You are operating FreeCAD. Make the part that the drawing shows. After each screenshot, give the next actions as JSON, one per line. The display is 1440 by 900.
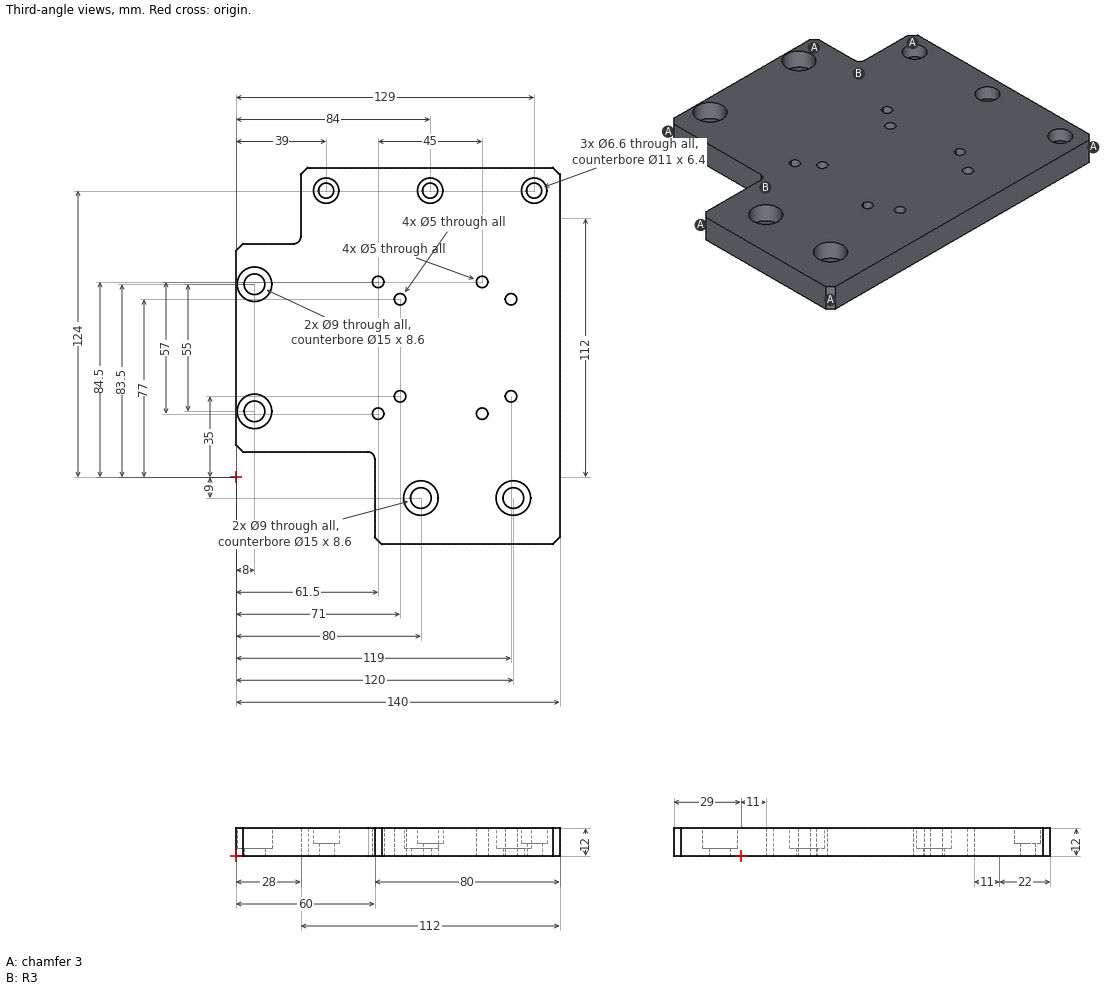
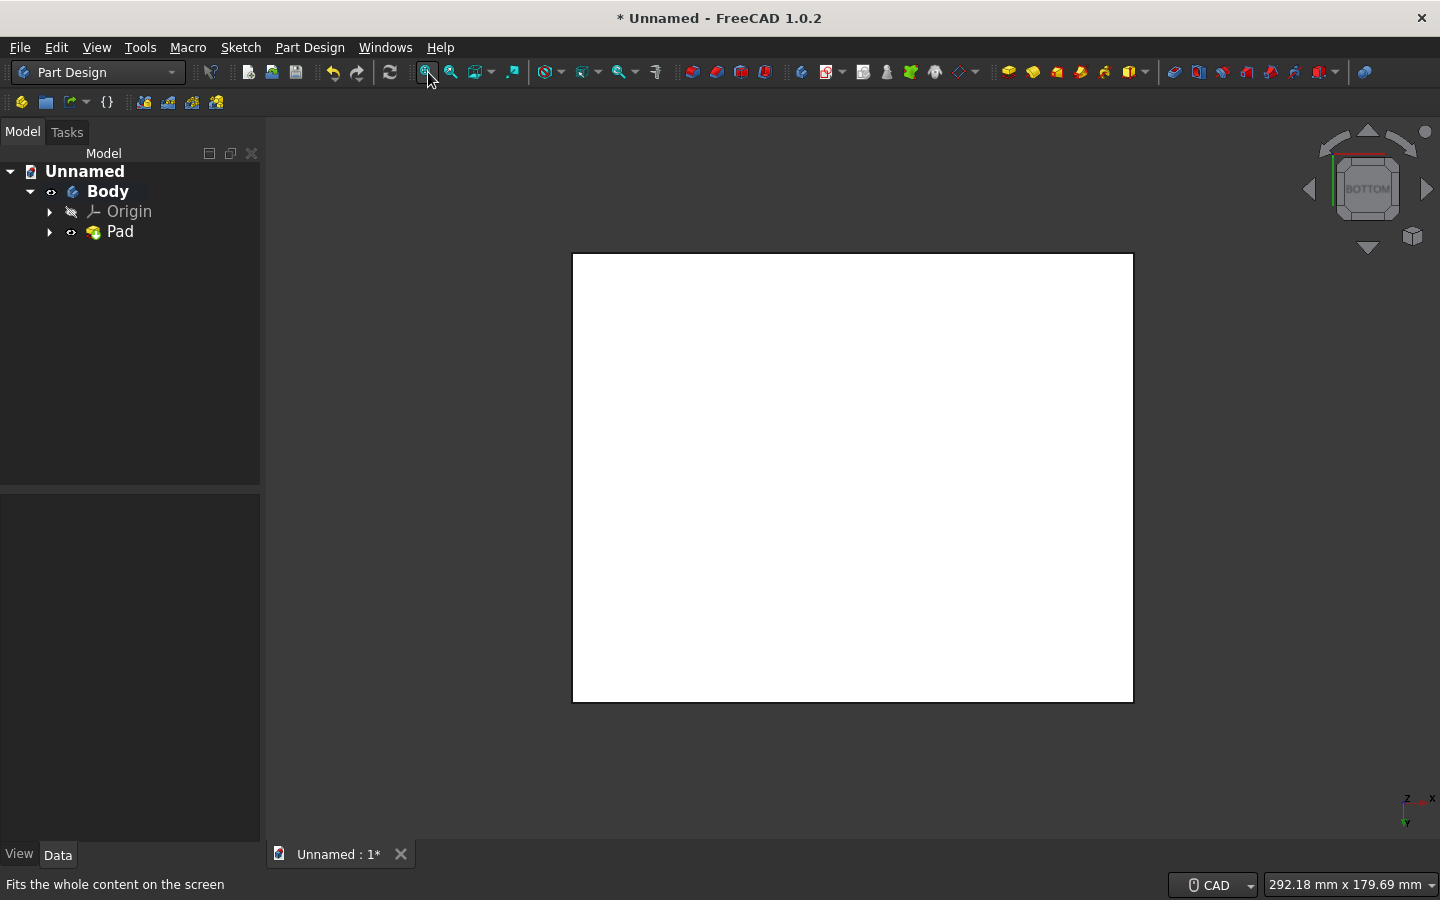
{"action": "left_click", "coordinate": [853, 477]}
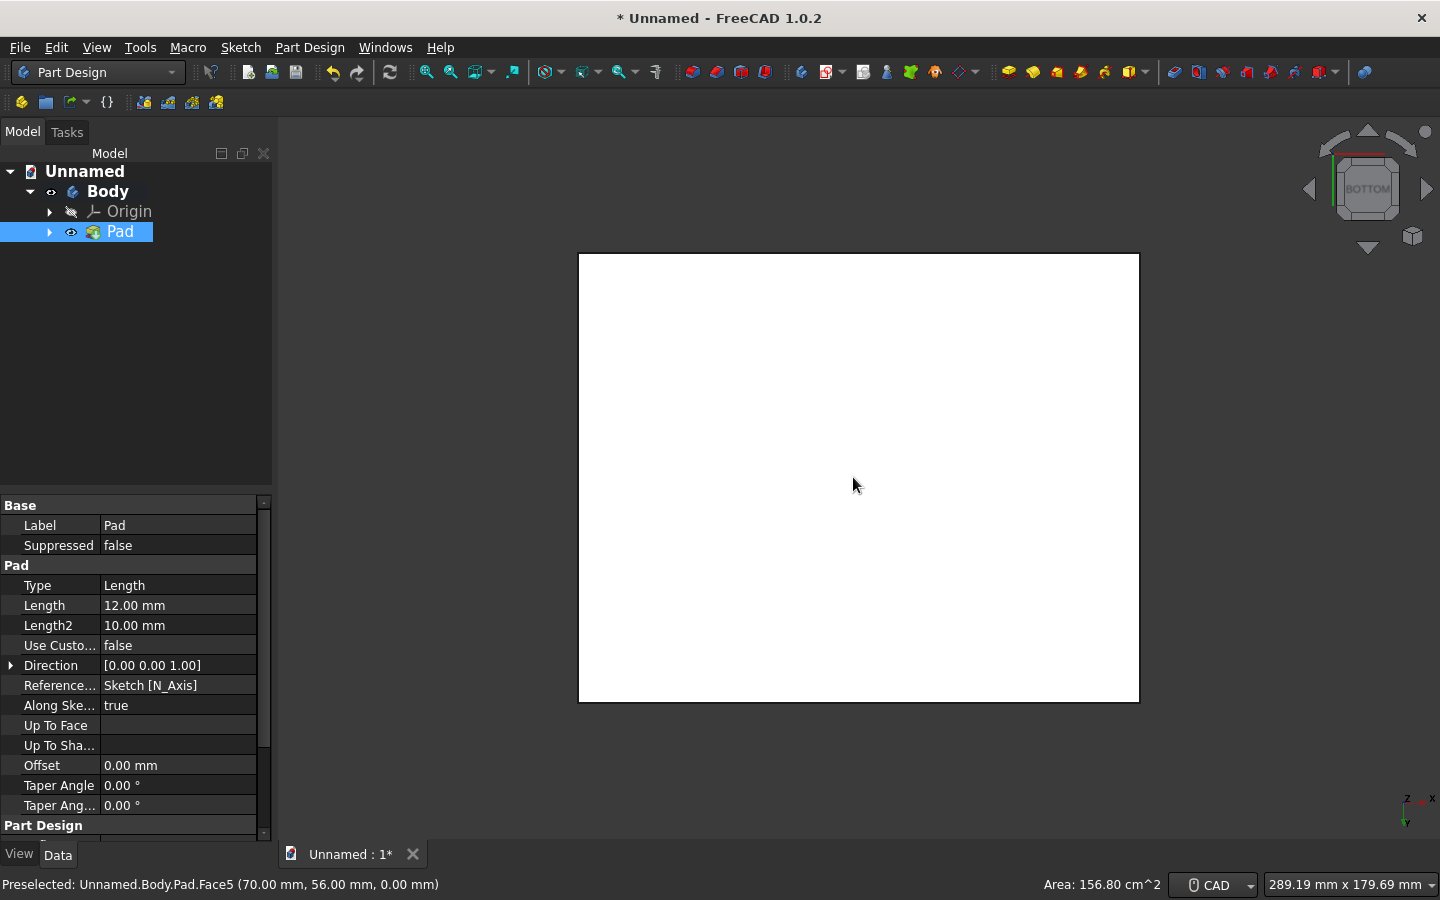
{"action": "left_click", "coordinate": [826, 72]}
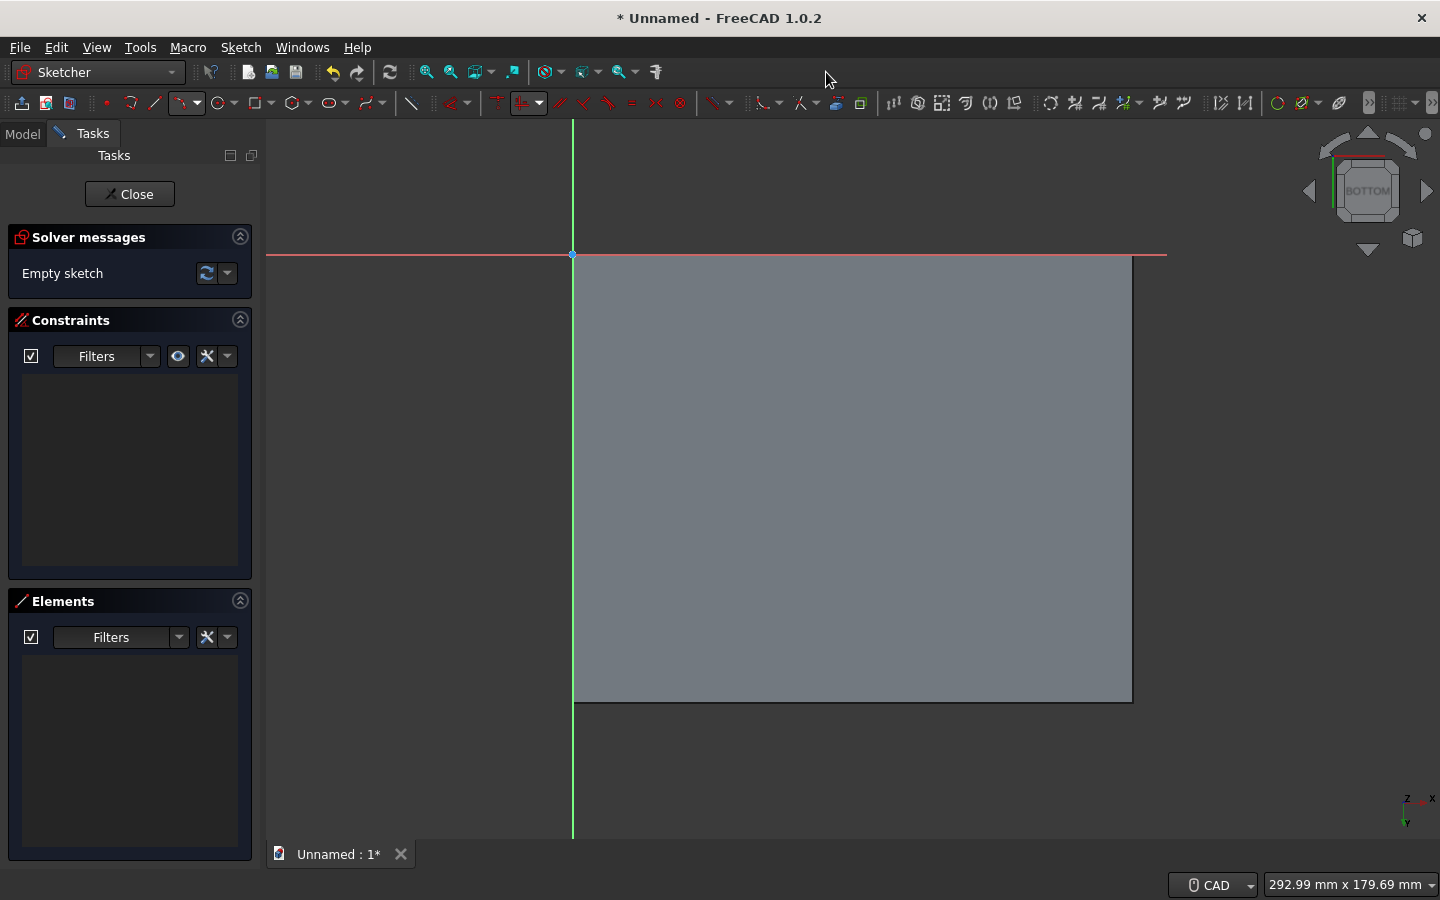
{"action": "left_click", "coordinate": [218, 104]}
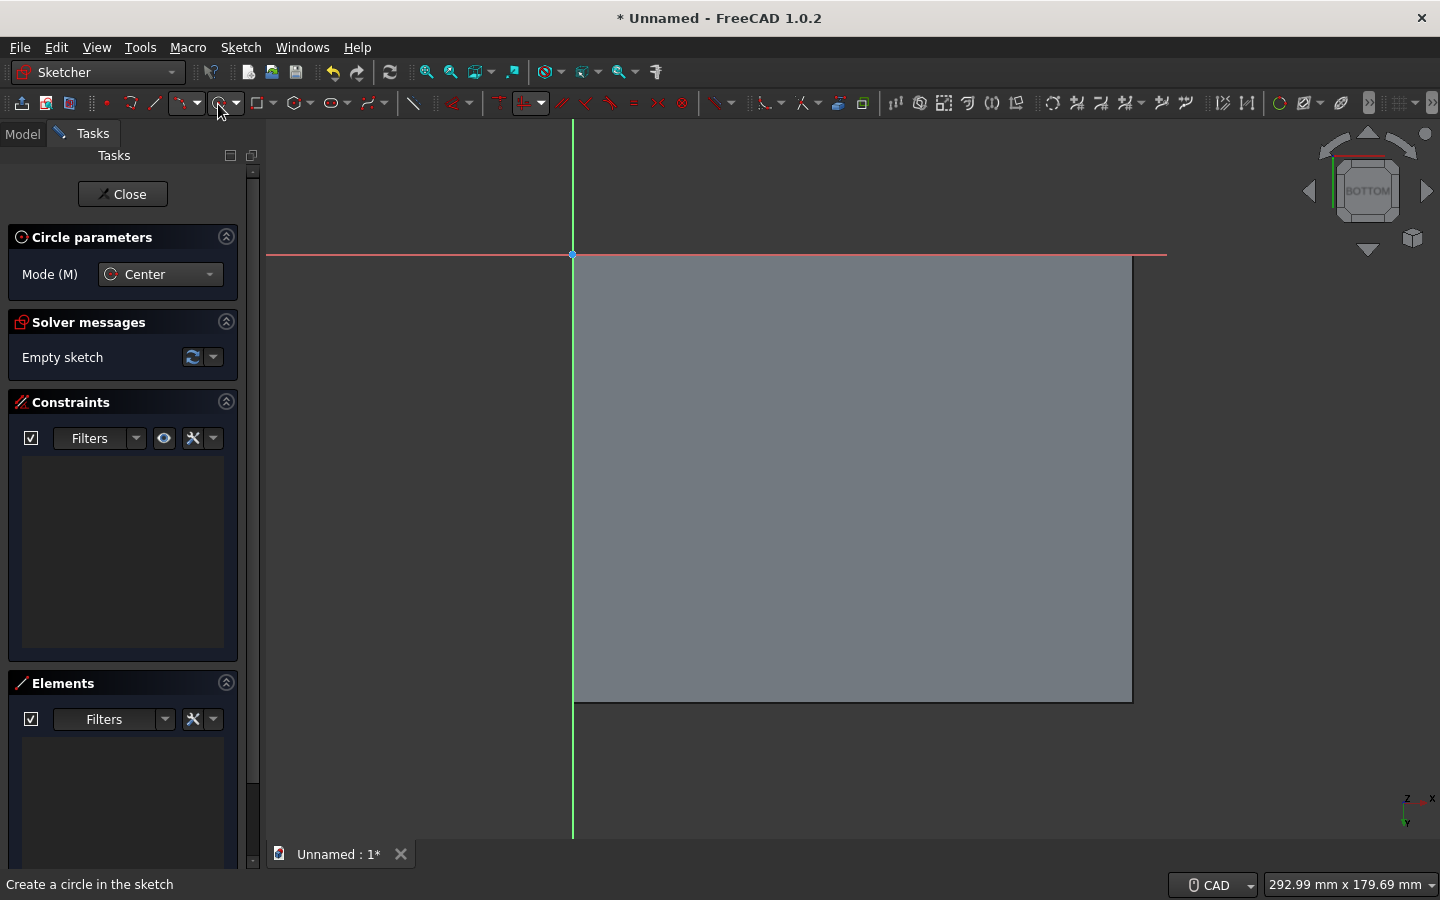
{"action": "scroll", "coordinate": [999, 593], "scroll_direction": "up", "scroll_amount": 5}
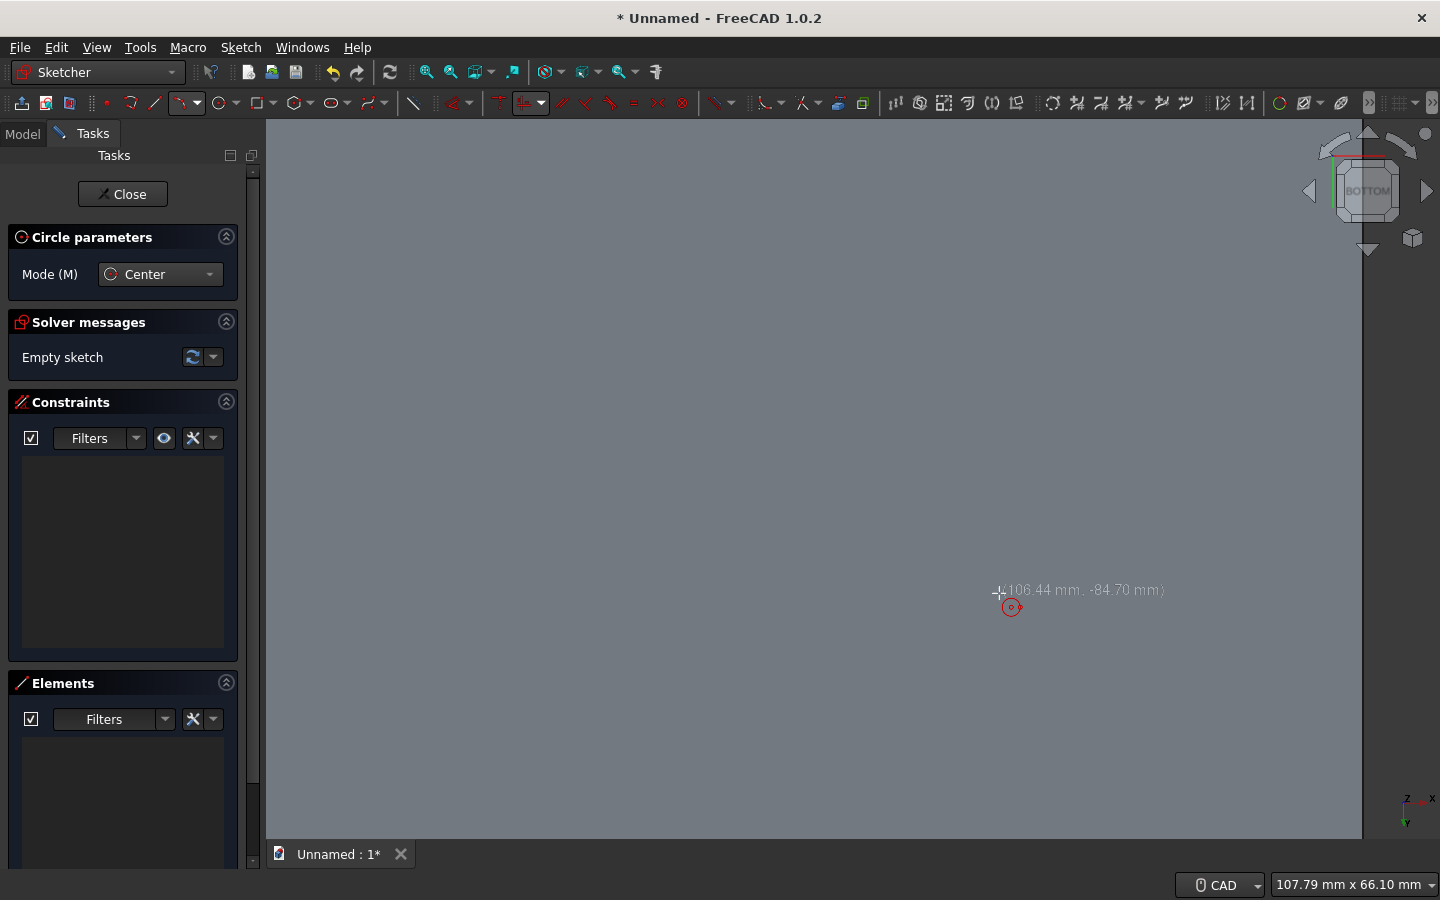
{"action": "left_click", "coordinate": [999, 592]}
{"action": "mouse_move", "coordinate": [1018, 573]}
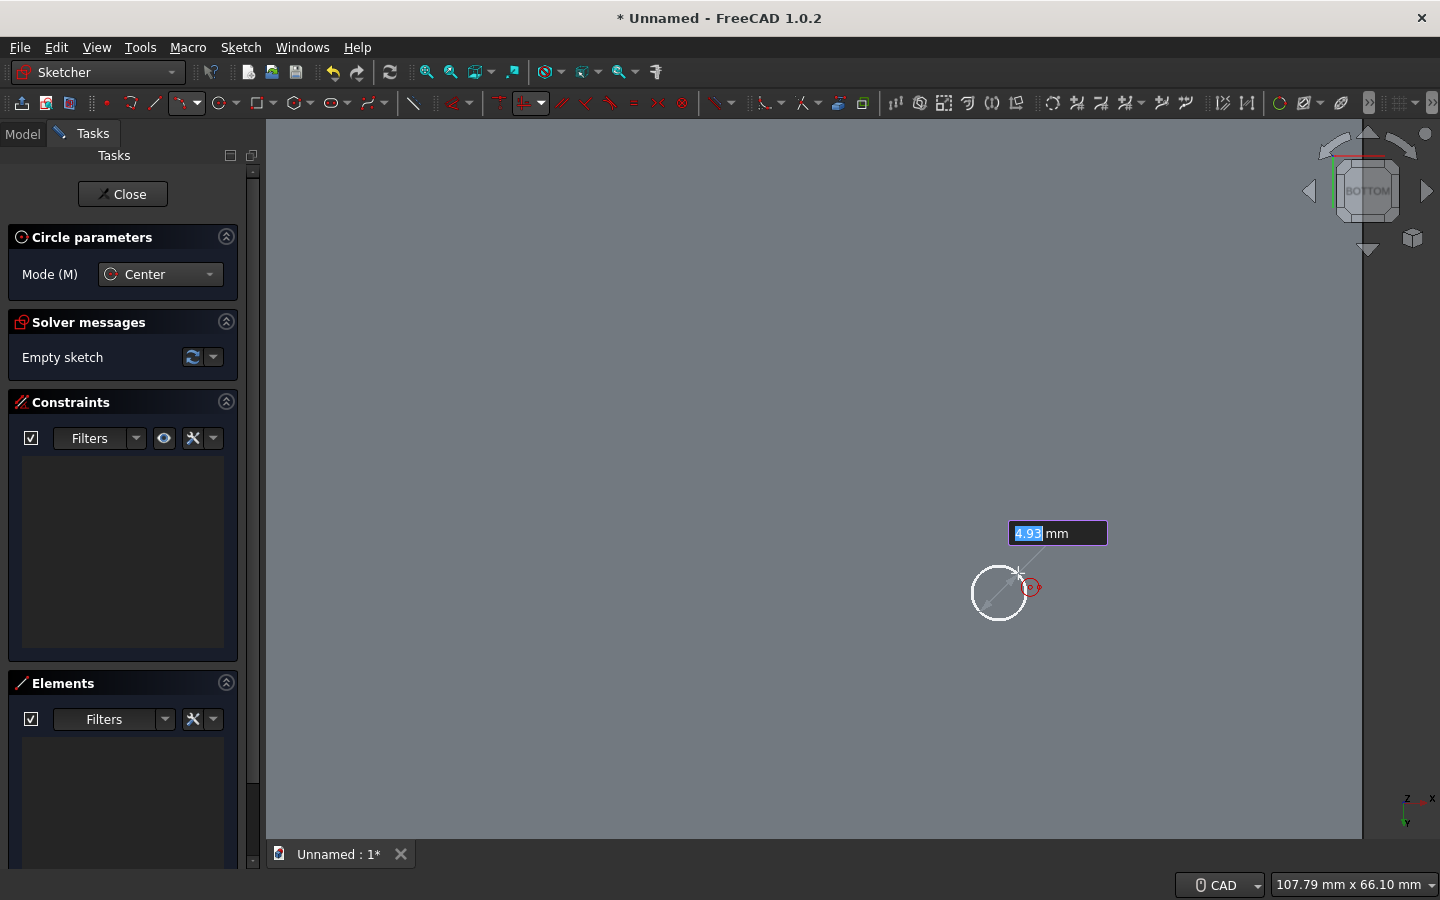
{"action": "type", "text": "5"}
{"action": "key", "text": "Return"}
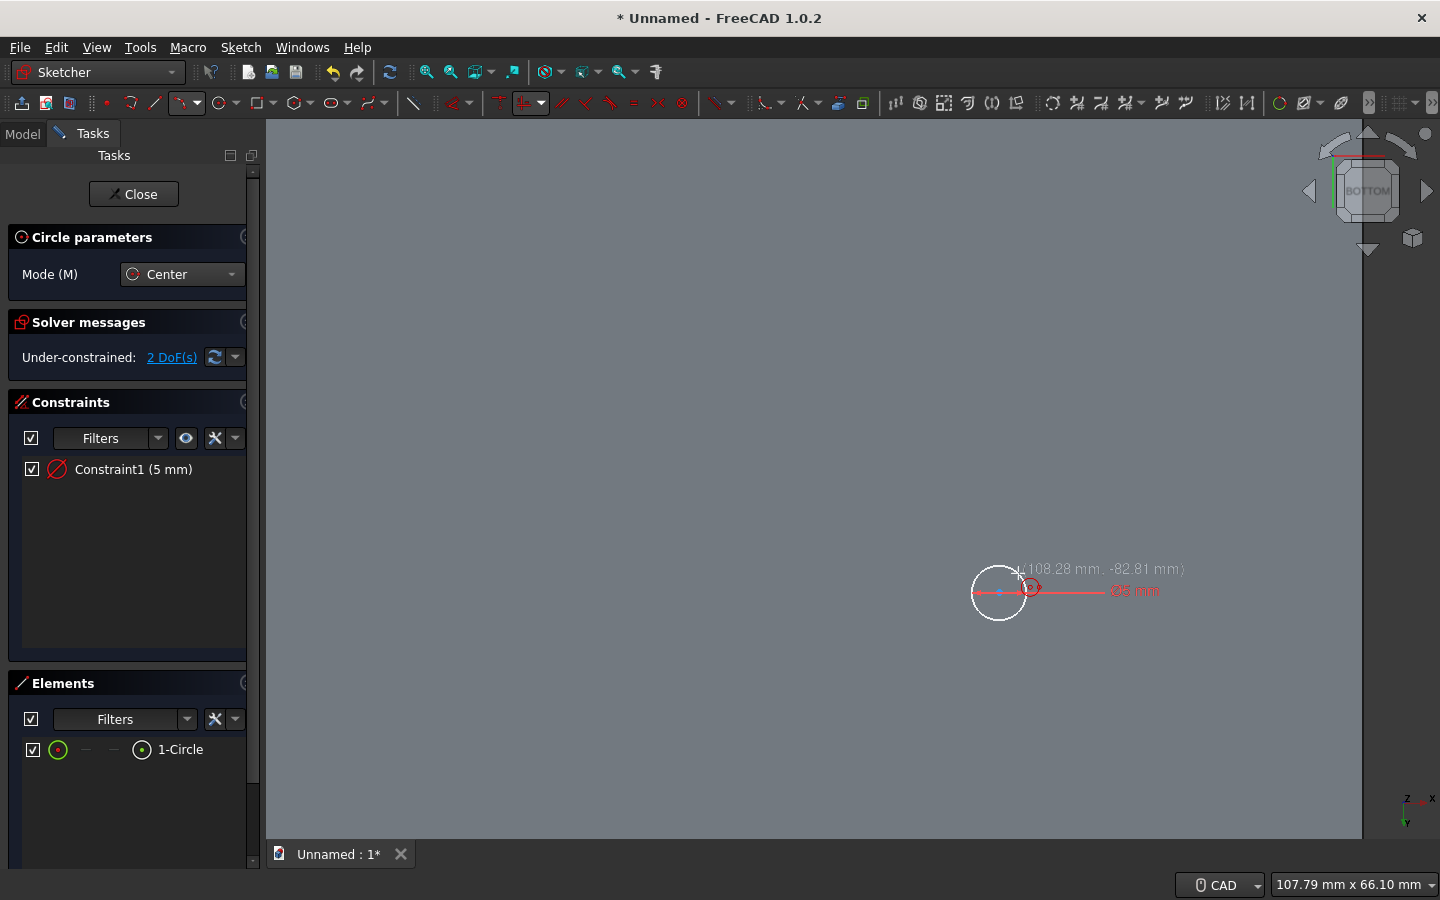
{"action": "left_click", "coordinate": [508, 592]}
{"action": "mouse_move", "coordinate": [528, 573]}